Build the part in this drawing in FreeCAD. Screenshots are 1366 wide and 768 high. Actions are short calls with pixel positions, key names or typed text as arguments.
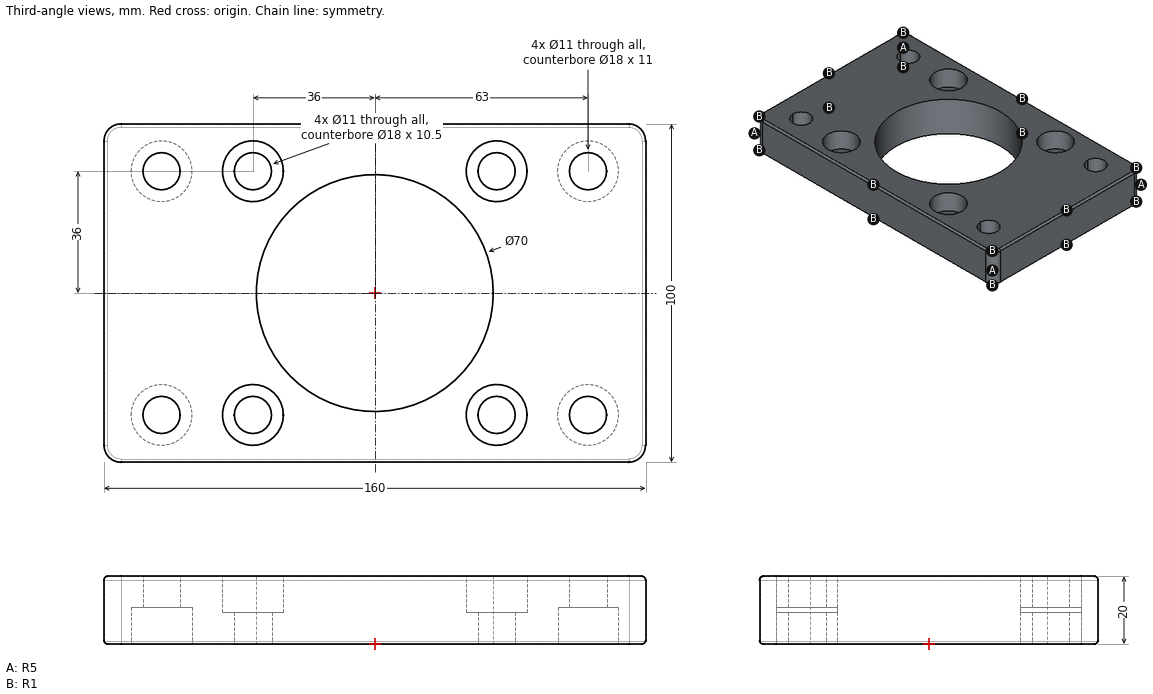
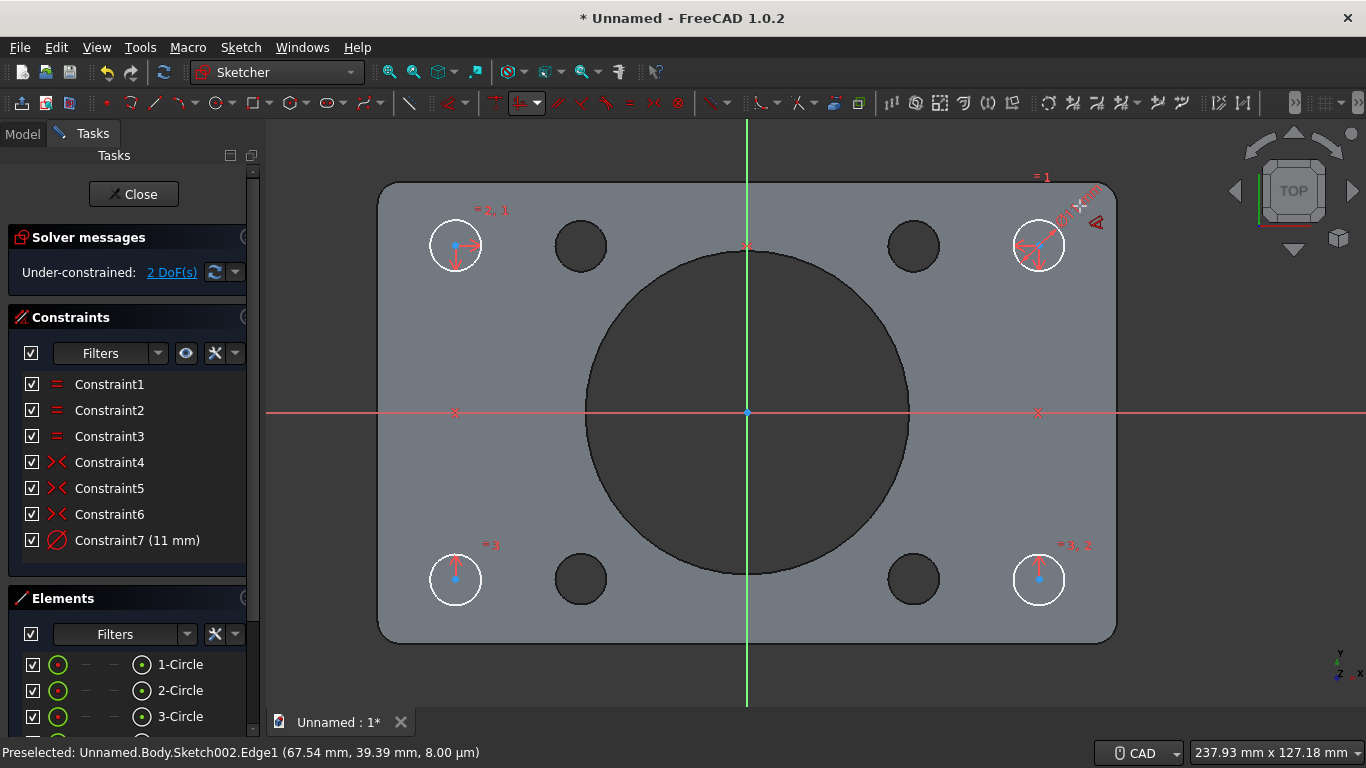
click(1039, 246)
click(893, 212)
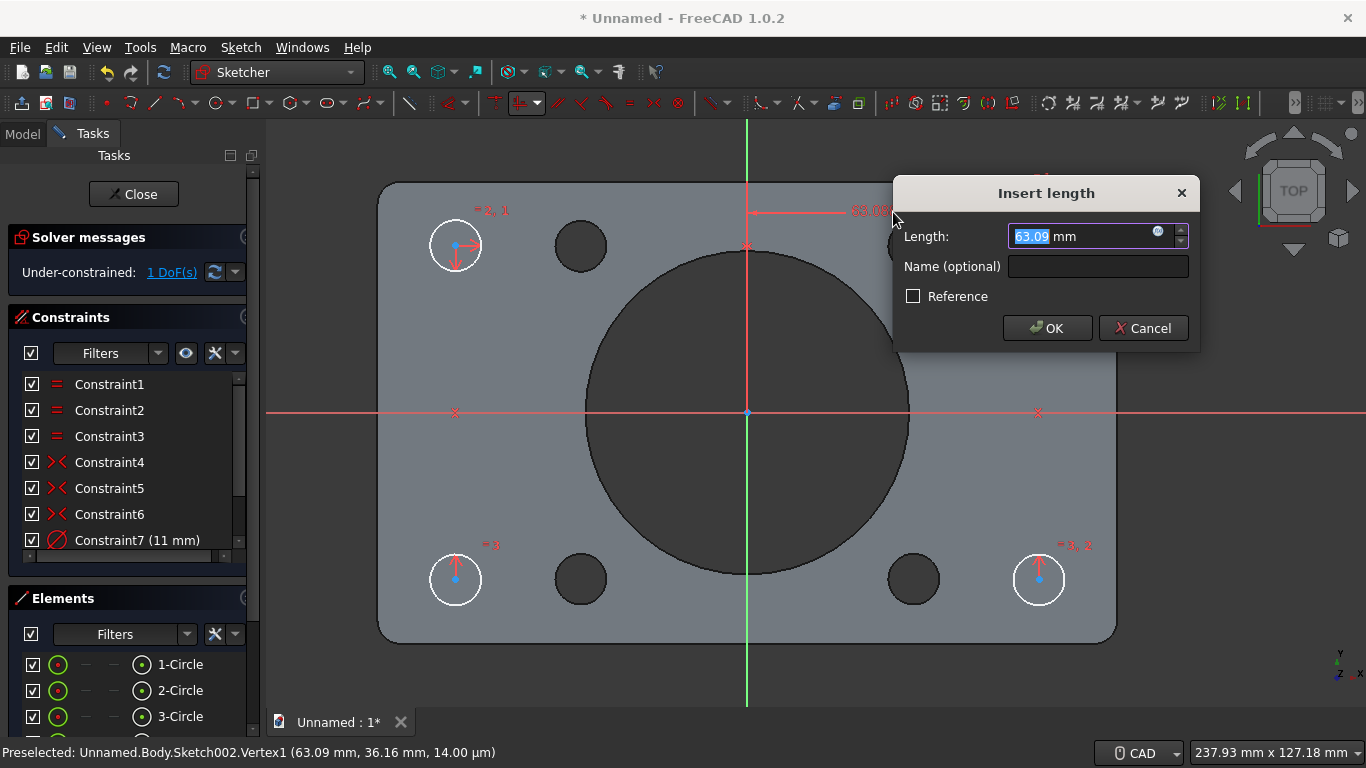
text(63)
key(Return)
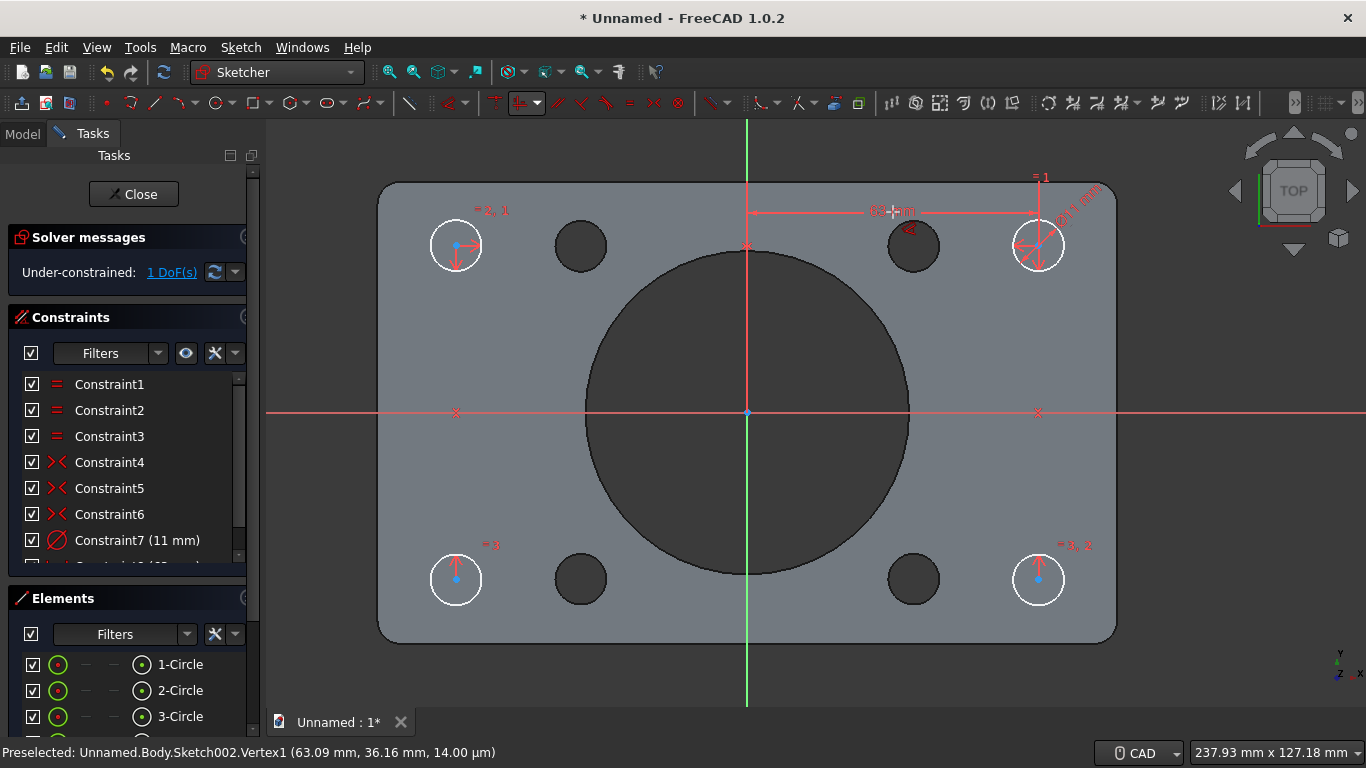
click(1039, 246)
click(1073, 329)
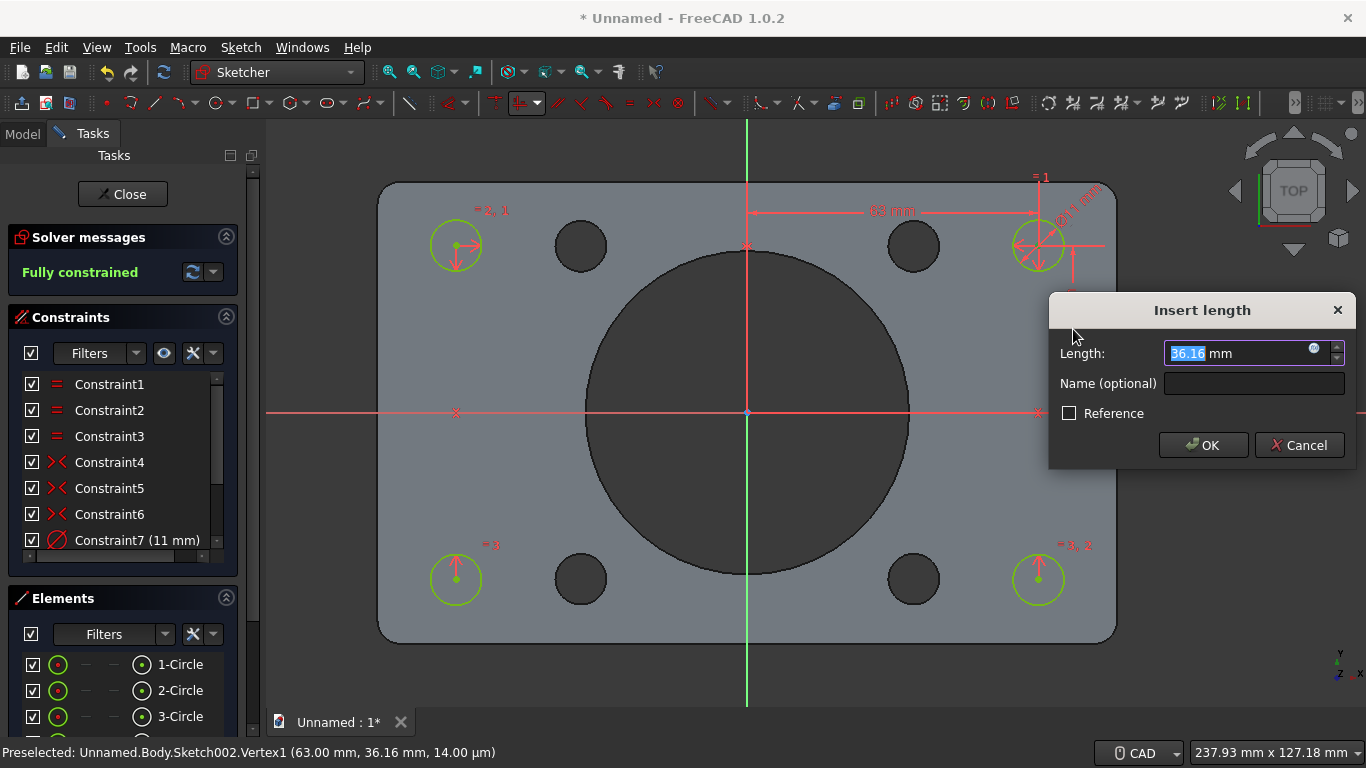
text(36)
key(Return)
key(Escape)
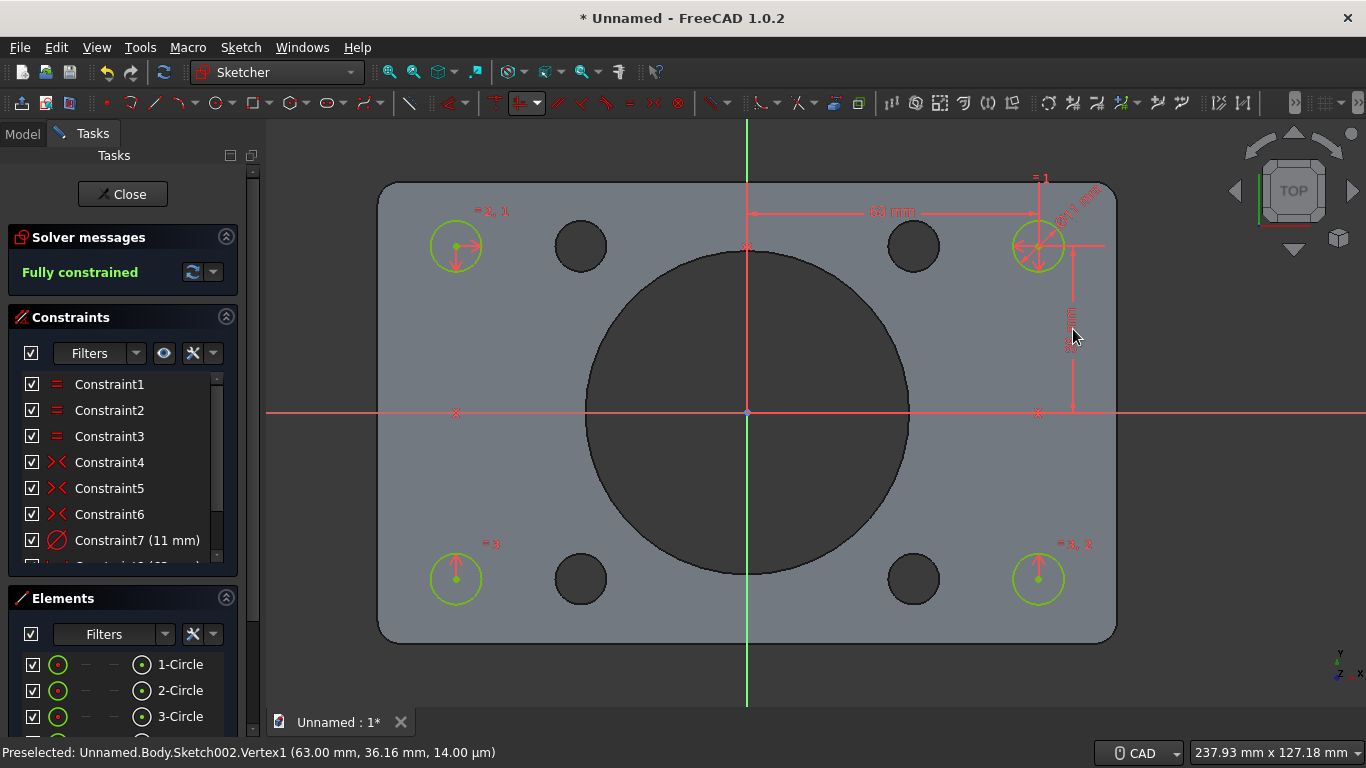
click(123, 194)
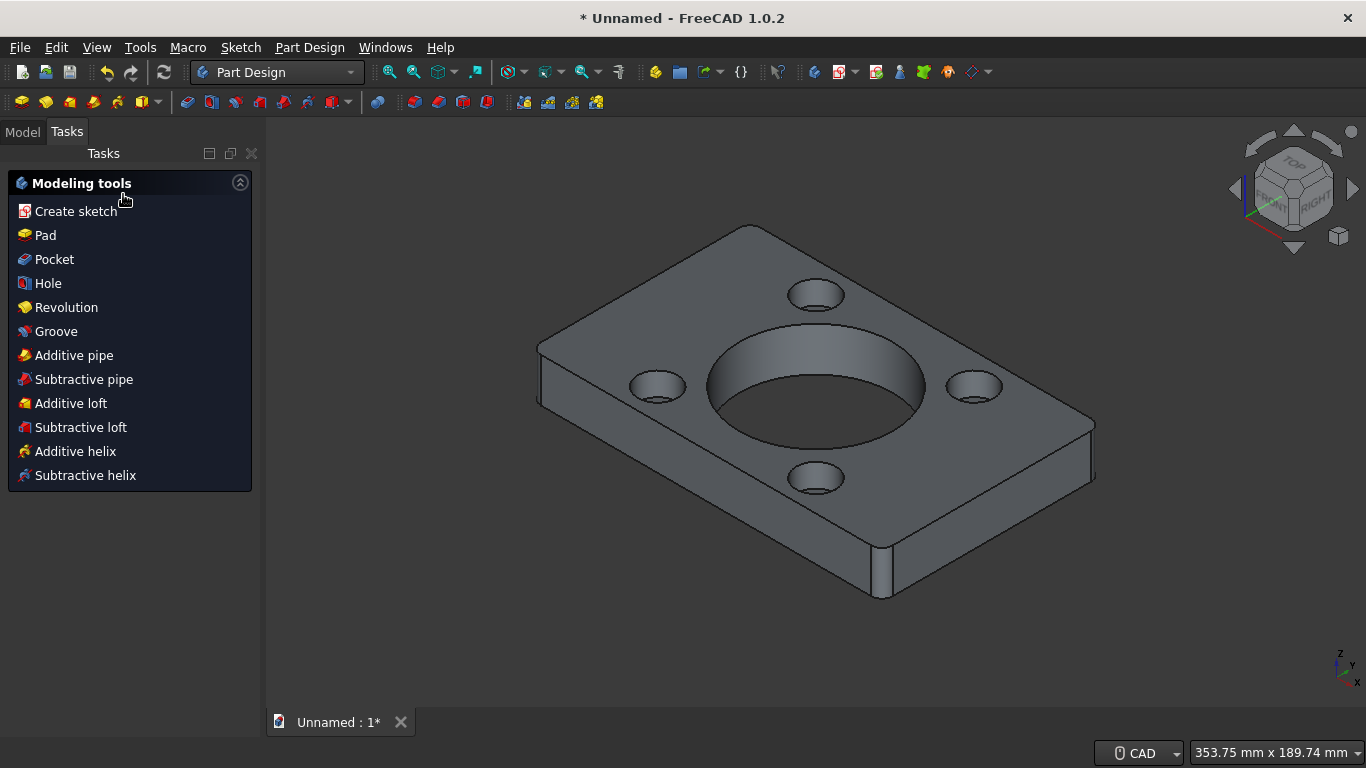
click(212, 102)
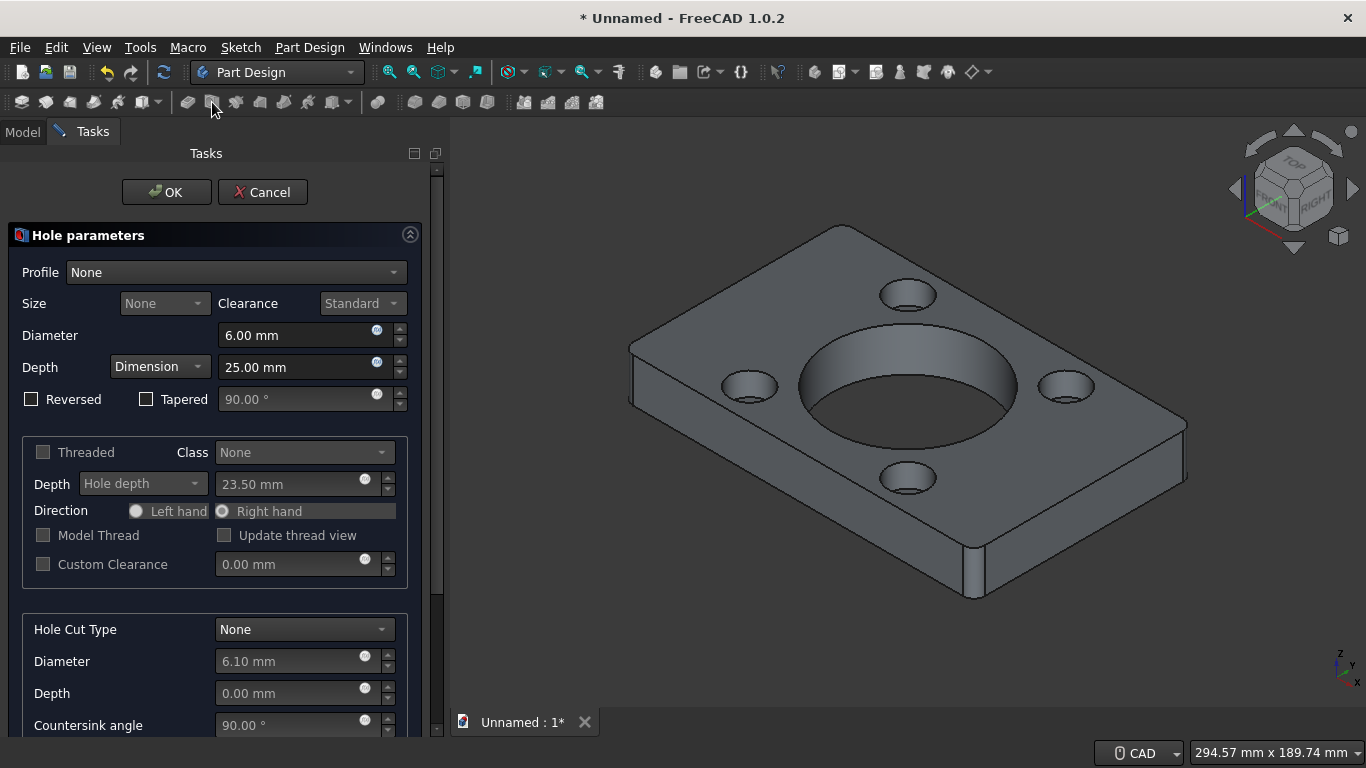
triple_click(305, 335)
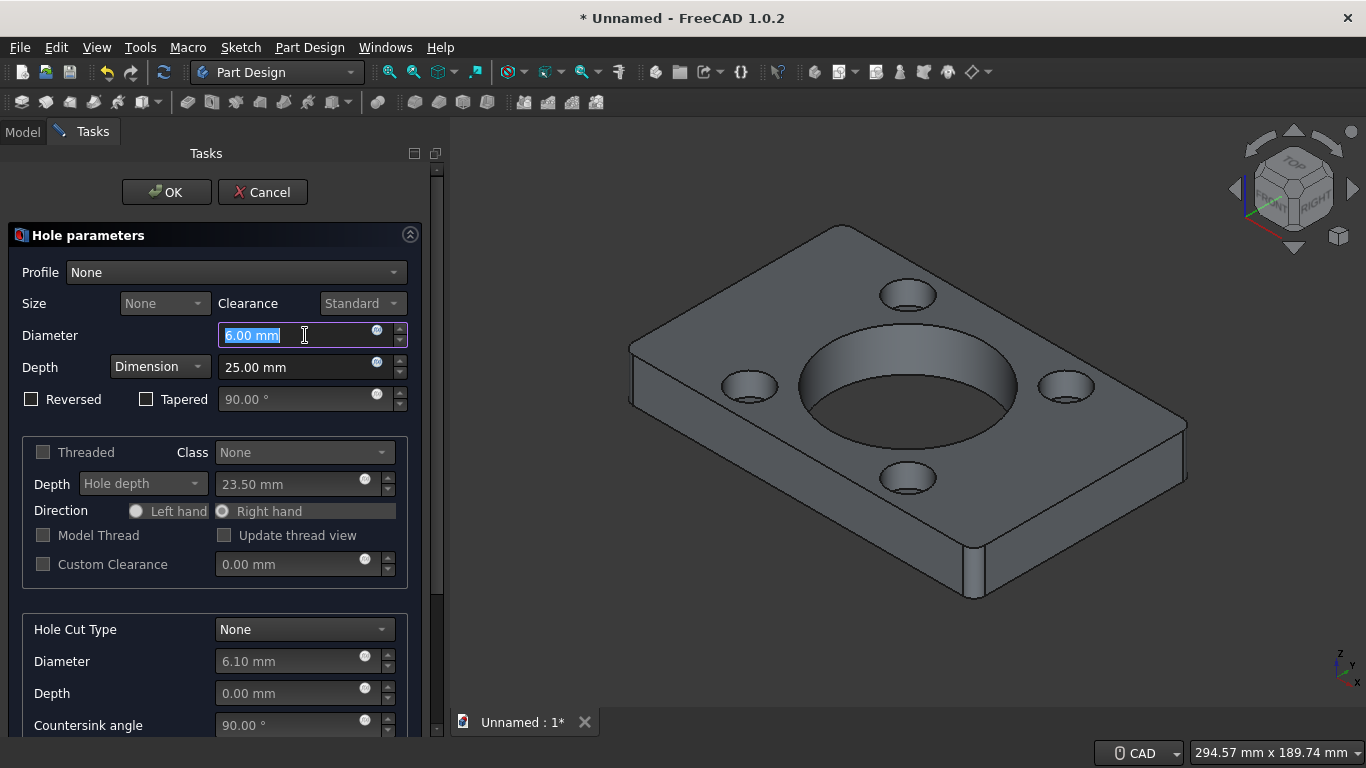
text(11)
key(Tab)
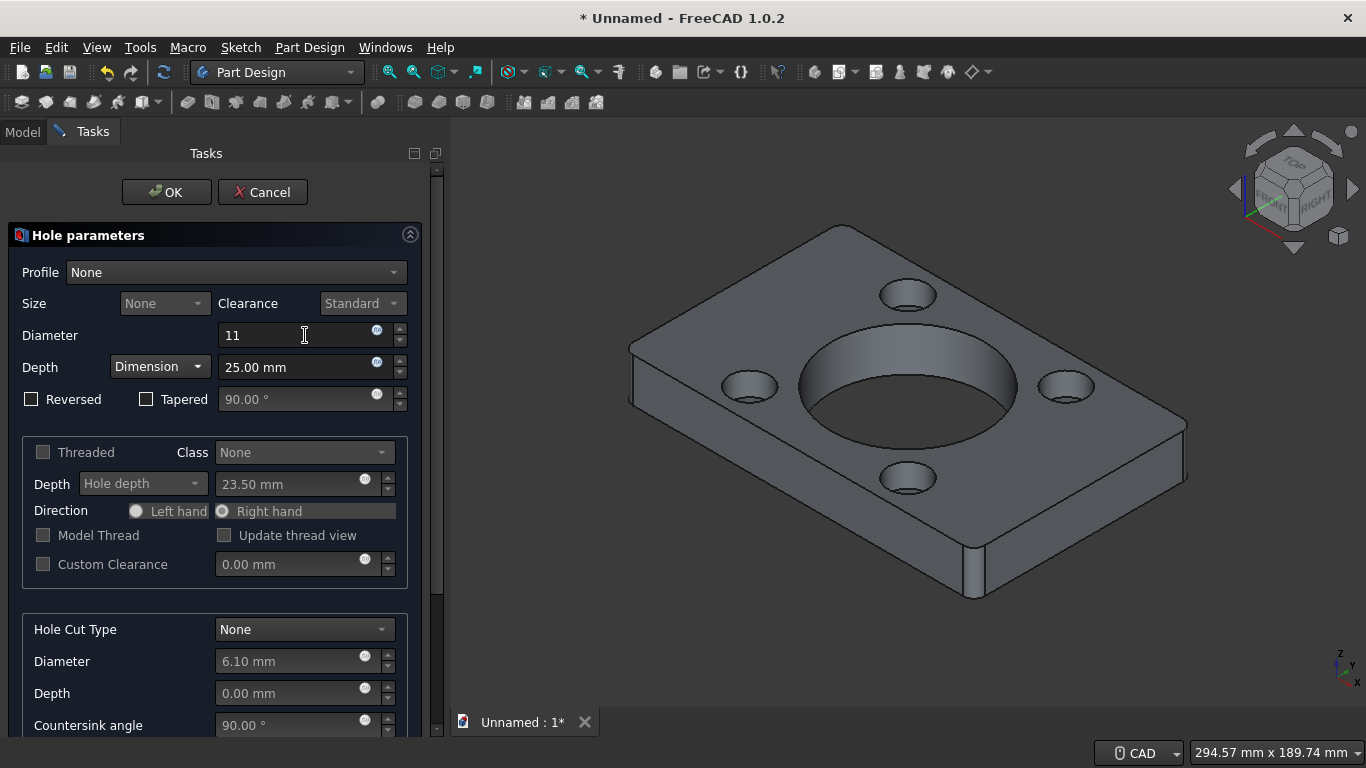
click(161, 366)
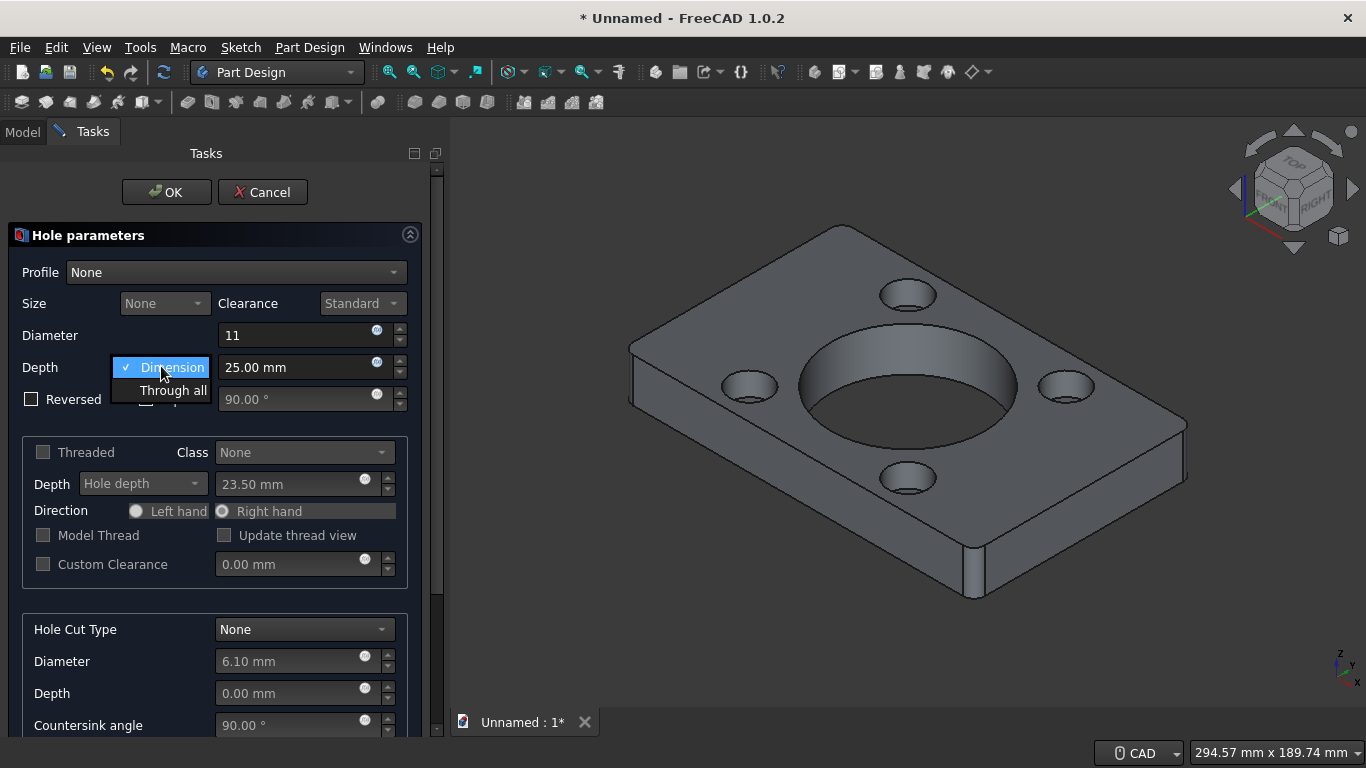
click(160, 390)